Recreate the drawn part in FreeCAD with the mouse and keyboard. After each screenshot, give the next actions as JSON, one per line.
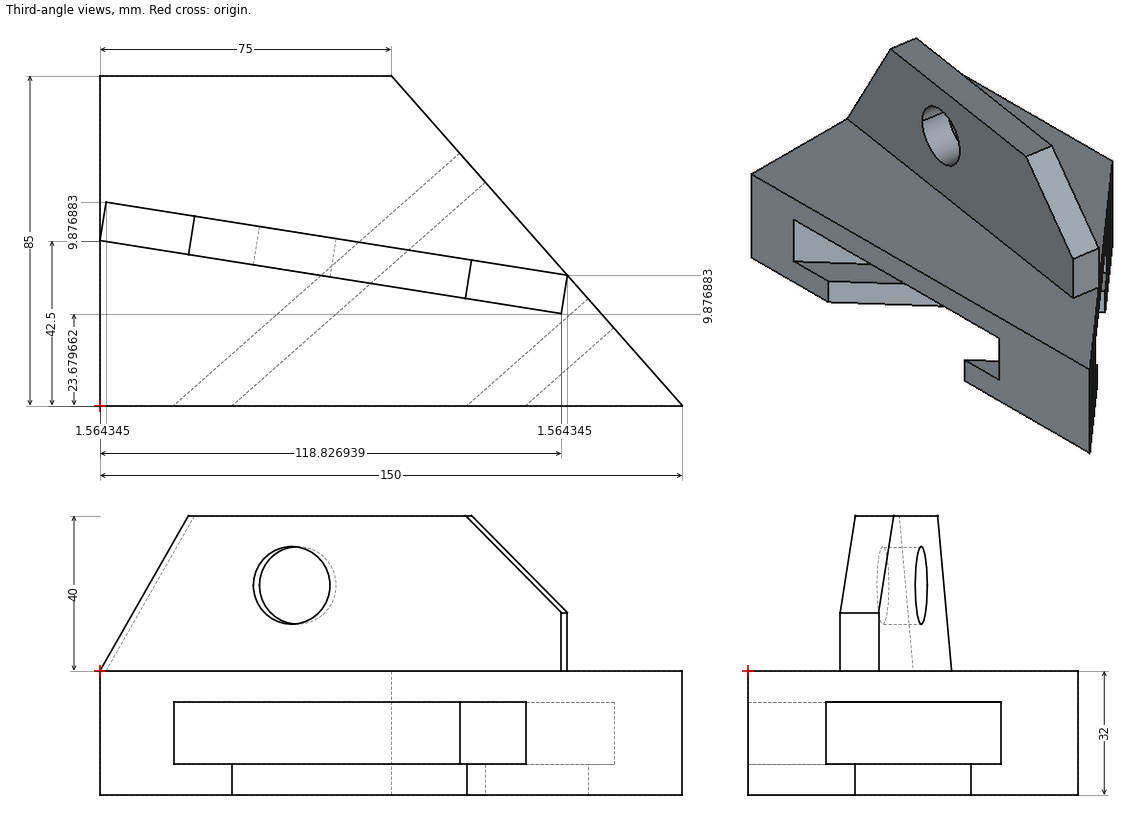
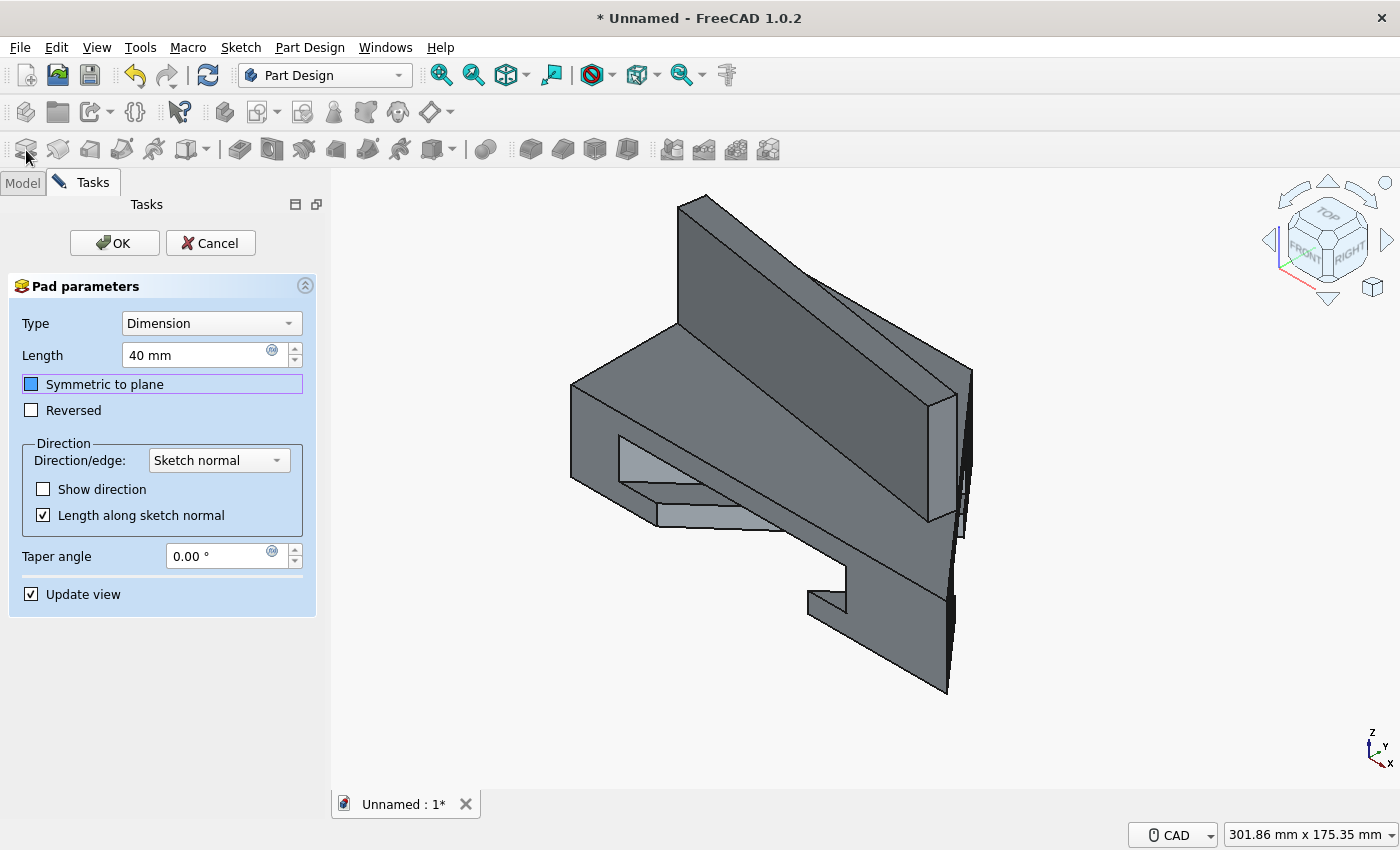
{"action": "left_click", "coordinate": [115, 243]}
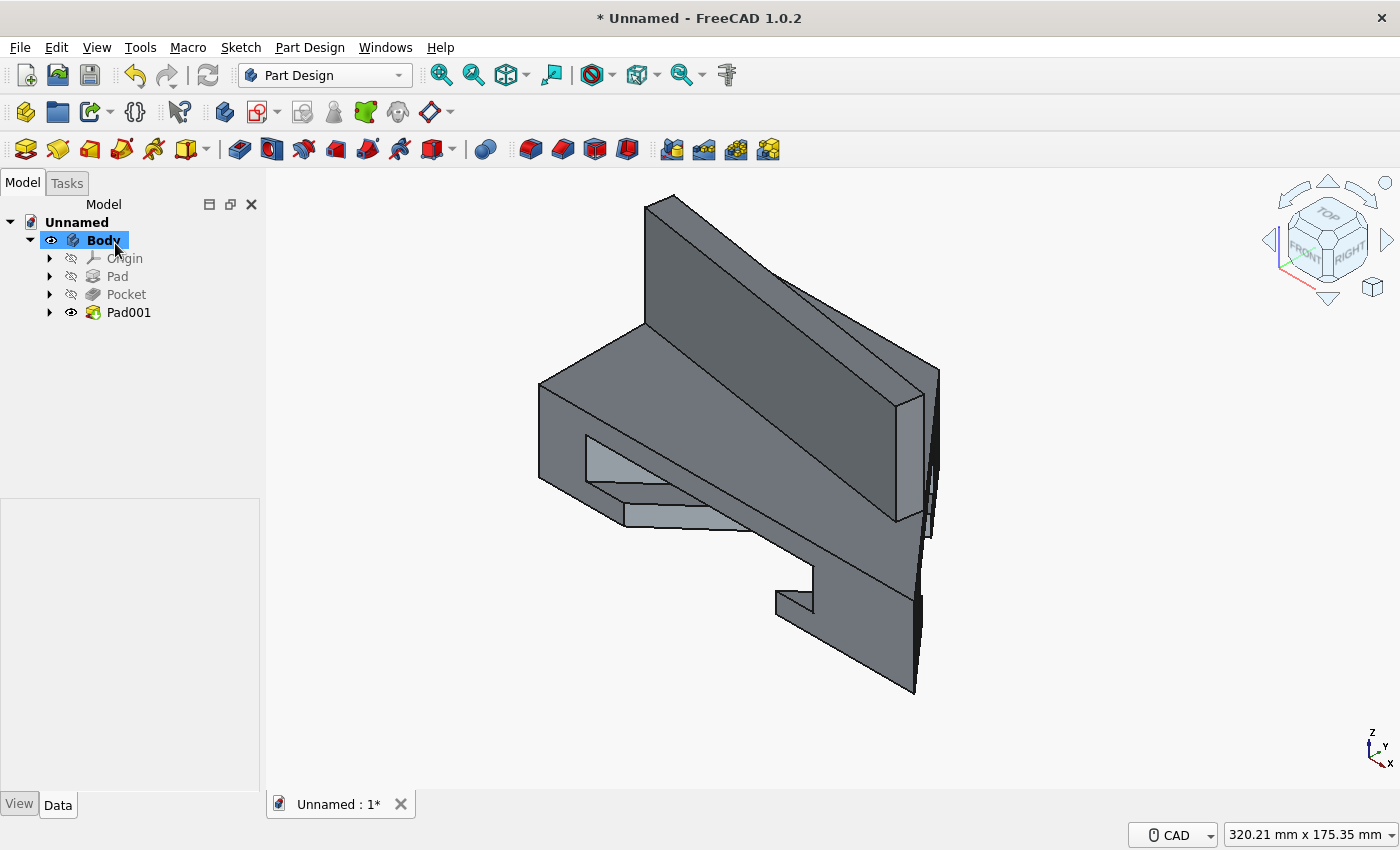
{"action": "key", "text": "v f"}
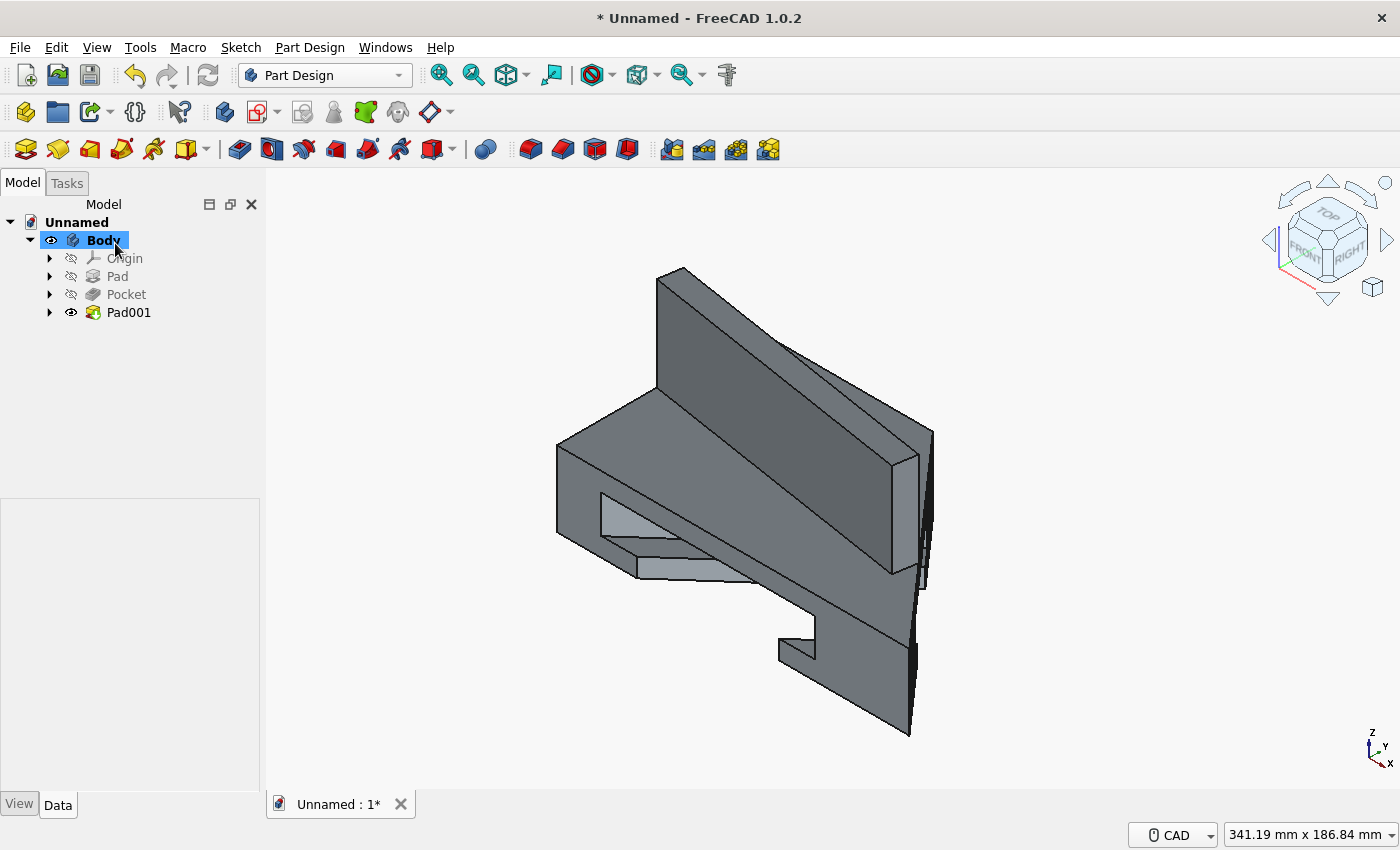
{"action": "key", "text": "4"}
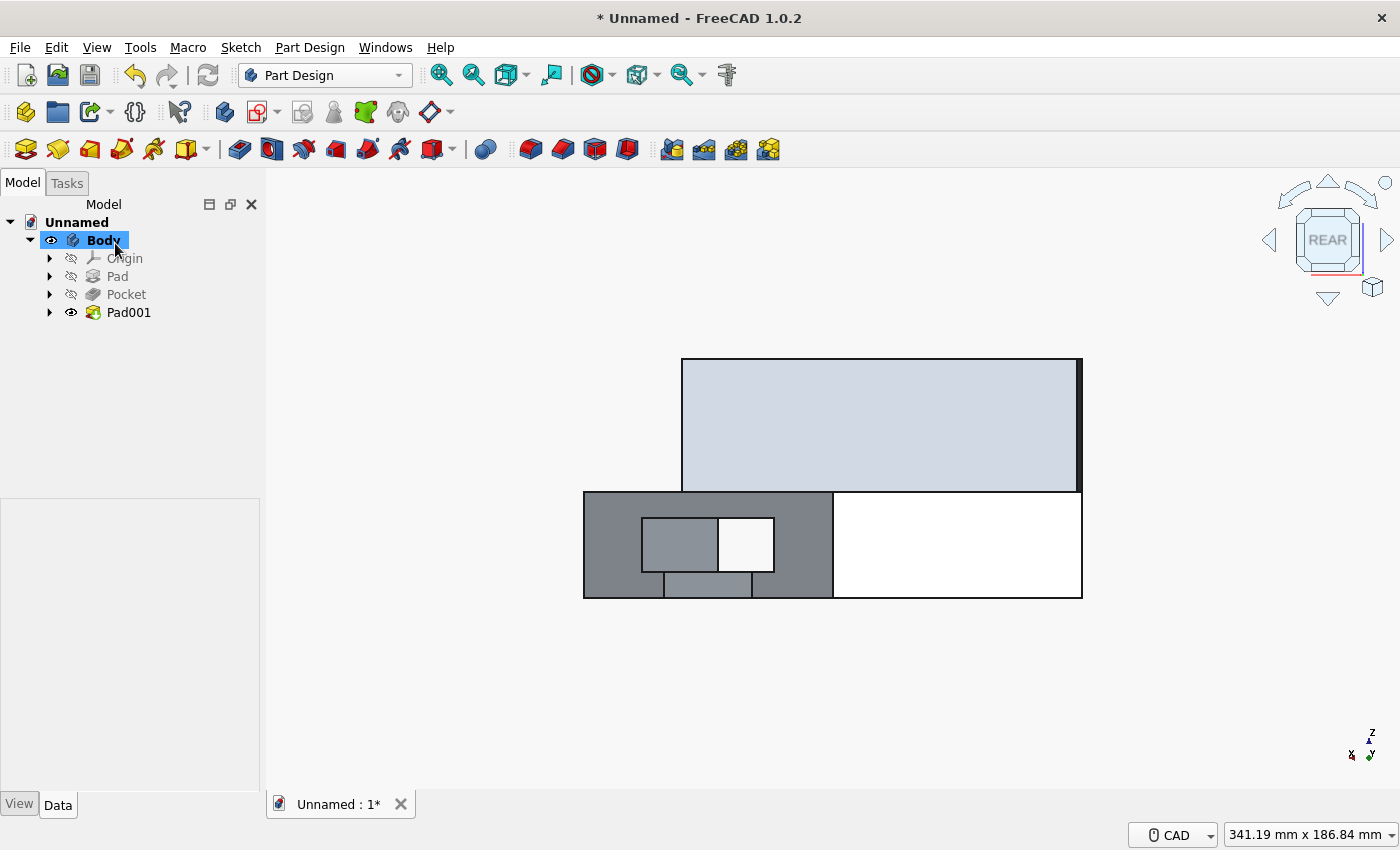
{"action": "key", "text": "v f"}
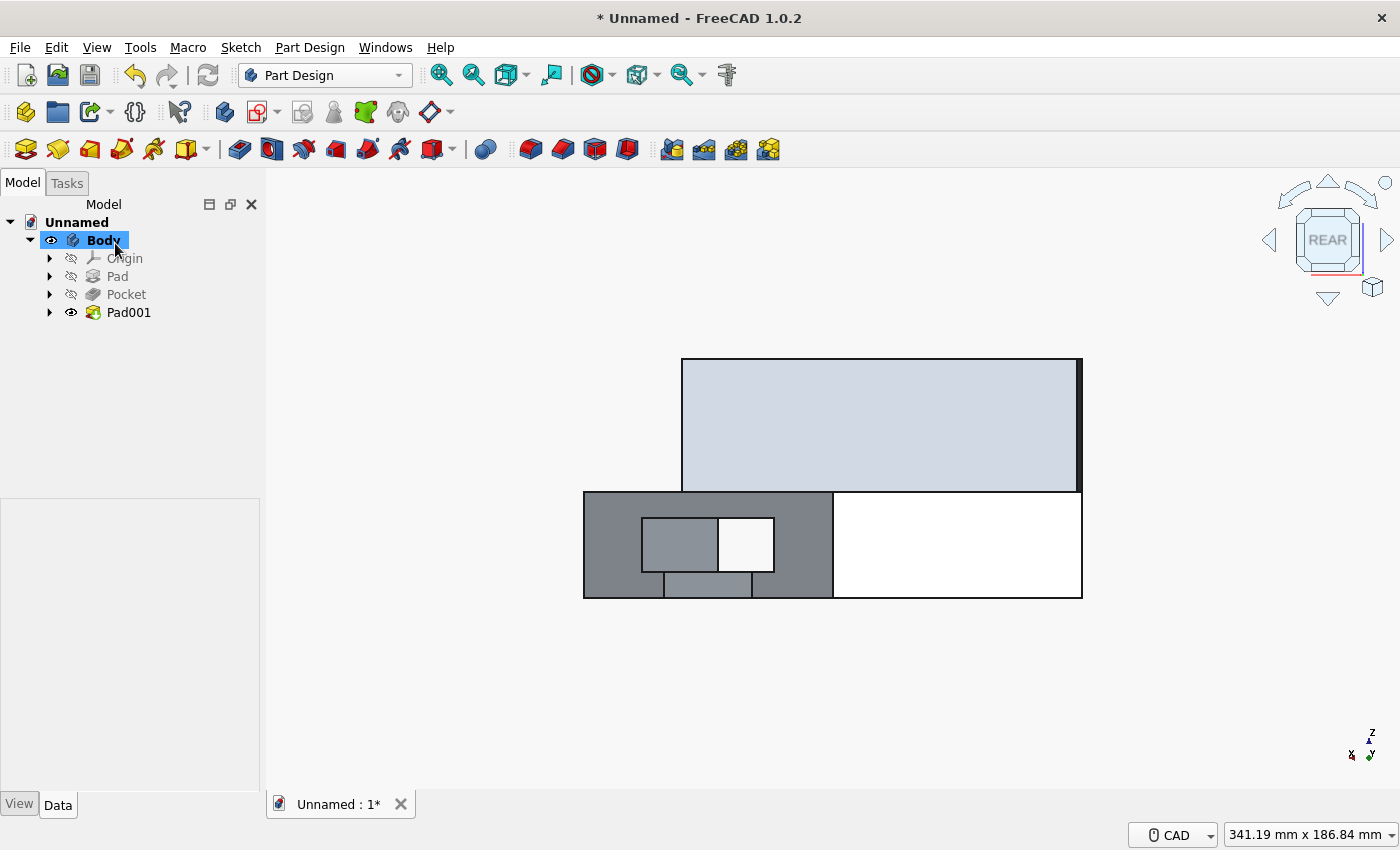
{"action": "left_click", "coordinate": [767, 424]}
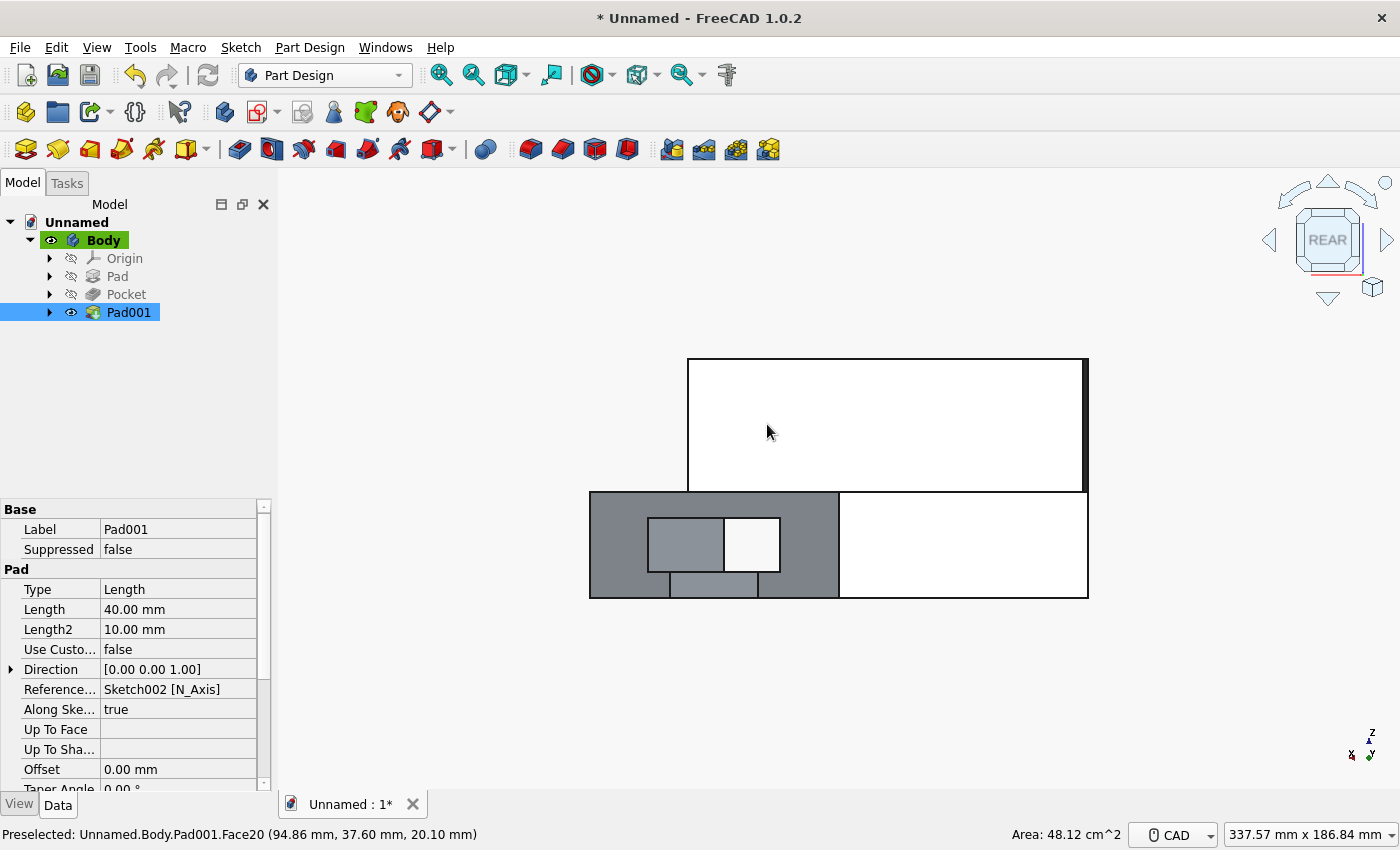
{"action": "left_click", "coordinate": [258, 112]}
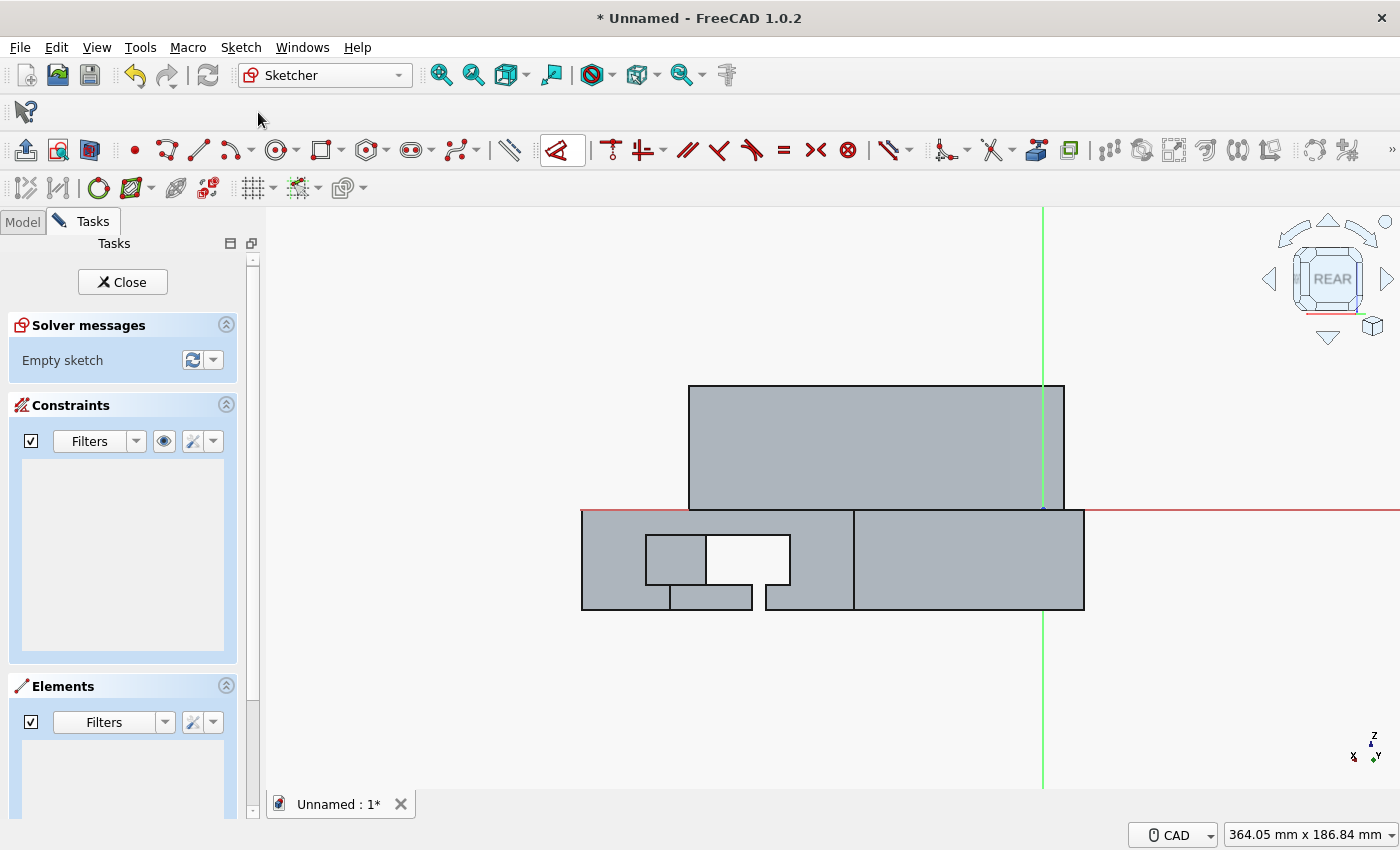
{"action": "key", "text": "q s"}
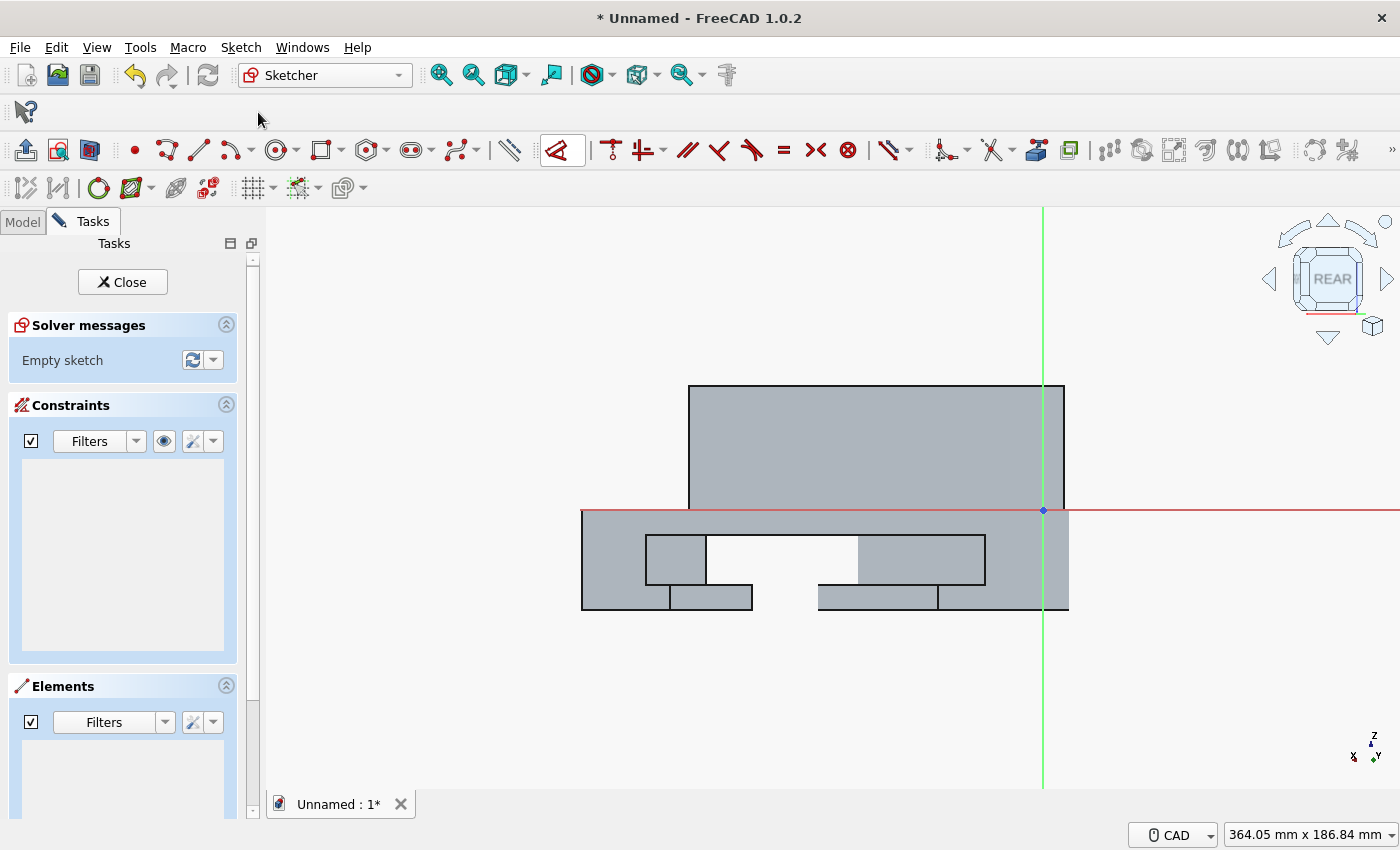
{"action": "scroll", "coordinate": [988, 313], "scroll_direction": "up", "scroll_amount": 2}